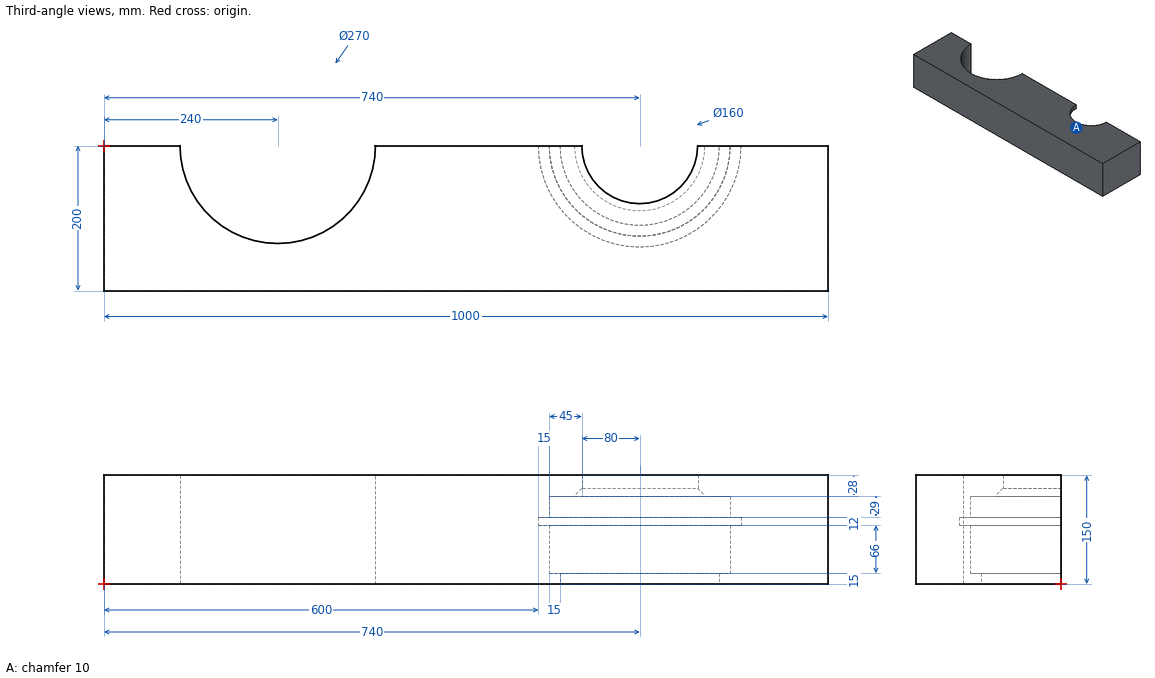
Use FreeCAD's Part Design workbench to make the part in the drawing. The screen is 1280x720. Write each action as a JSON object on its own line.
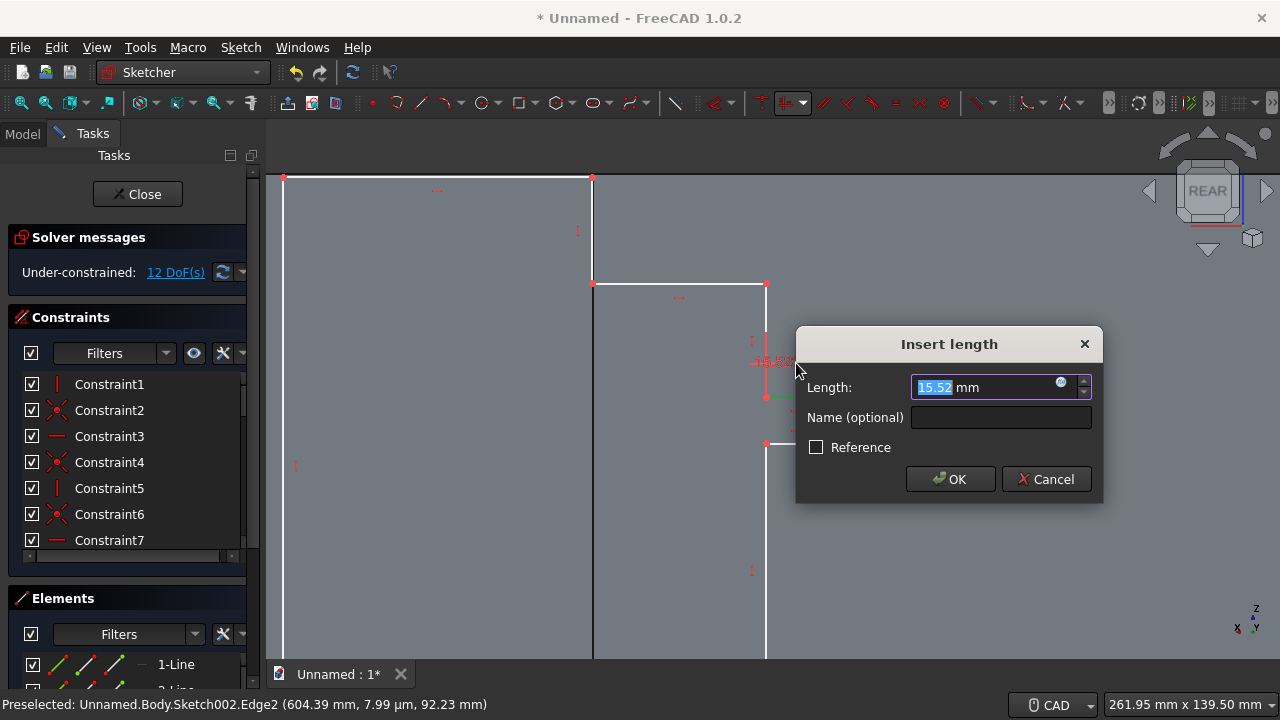
{"action": "type", "text": "15"}
{"action": "key", "text": "Return"}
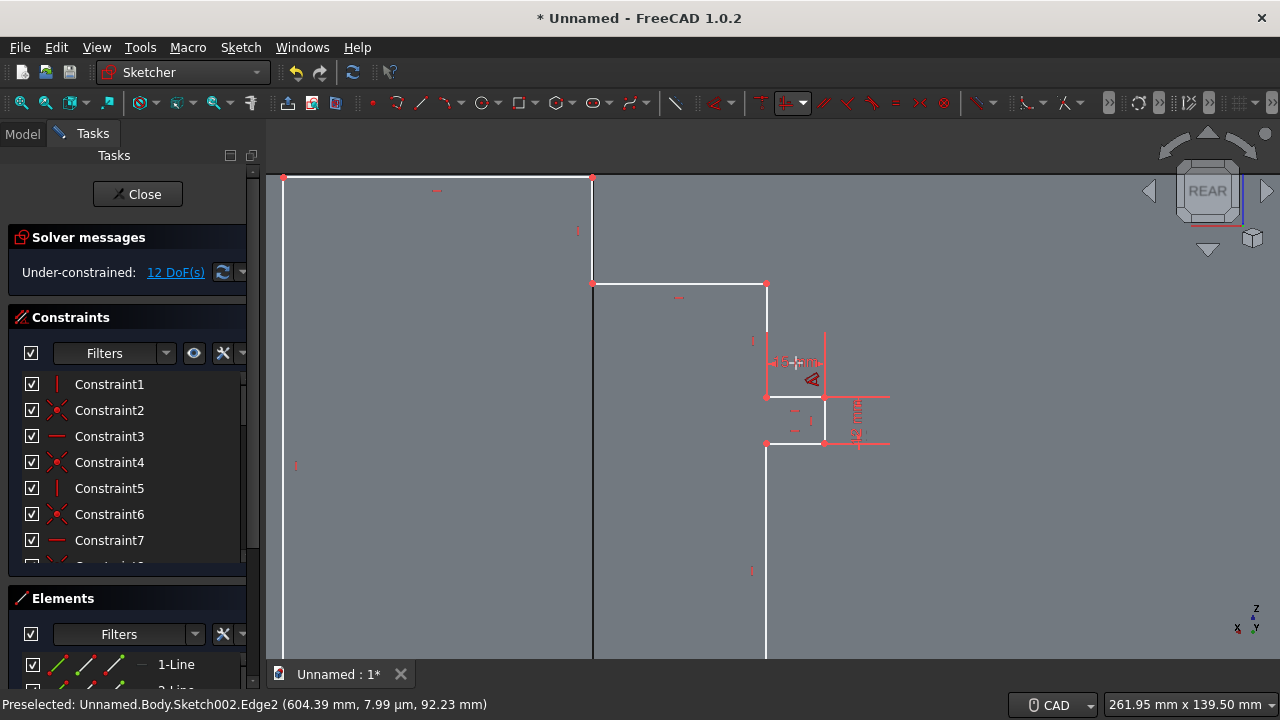
{"action": "left_click", "coordinate": [767, 363]}
{"action": "left_click", "coordinate": [801, 341]}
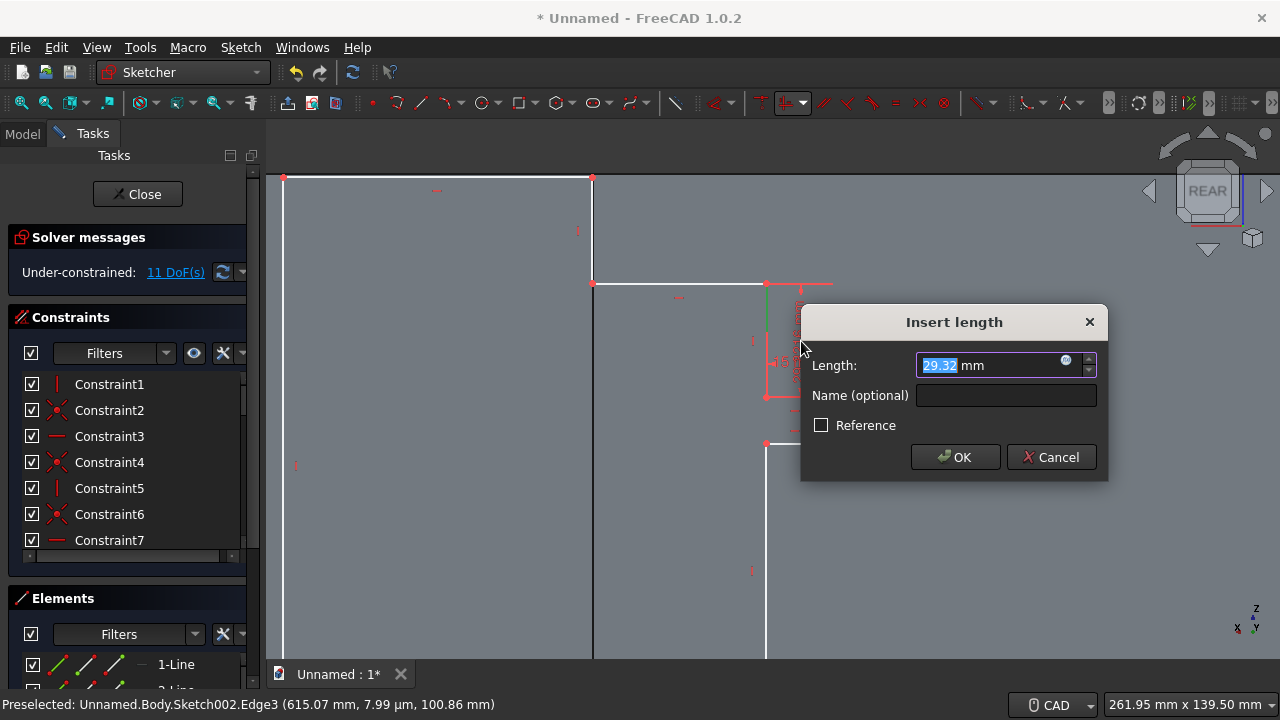
{"action": "type", "text": "29"}
{"action": "key", "text": "Return"}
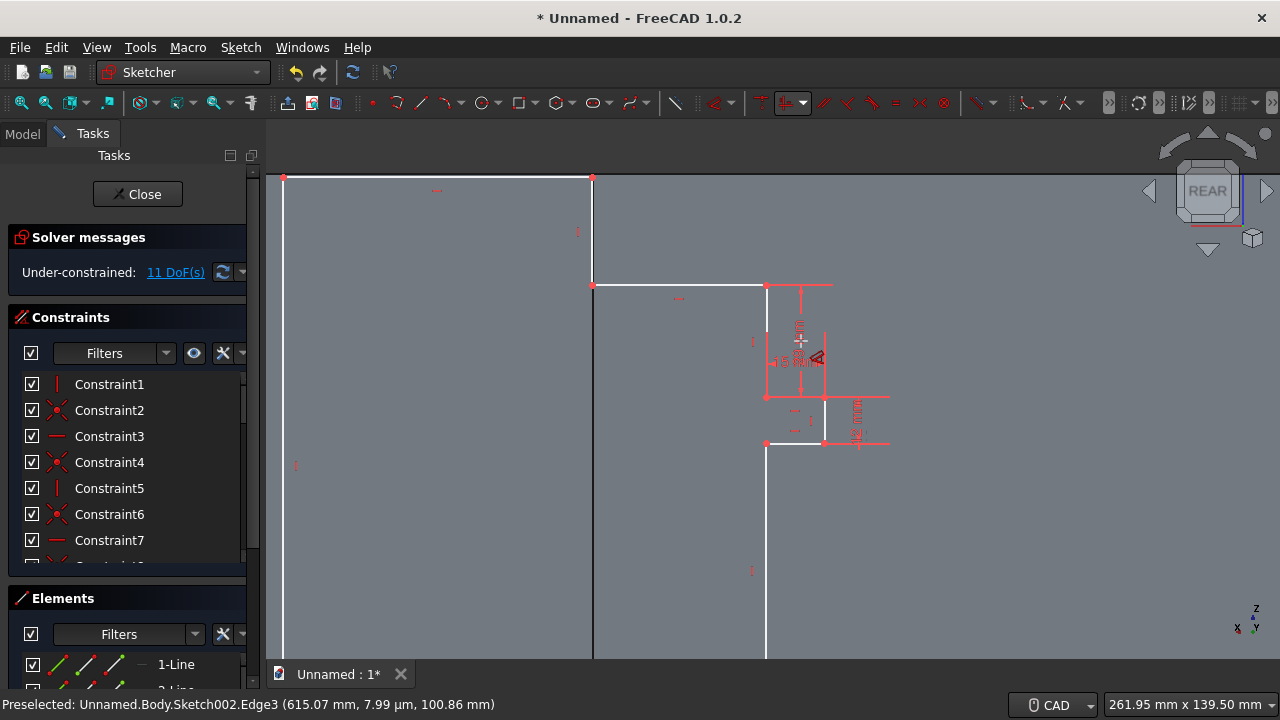
{"action": "left_click", "coordinate": [714, 285]}
{"action": "left_click", "coordinate": [680, 251]}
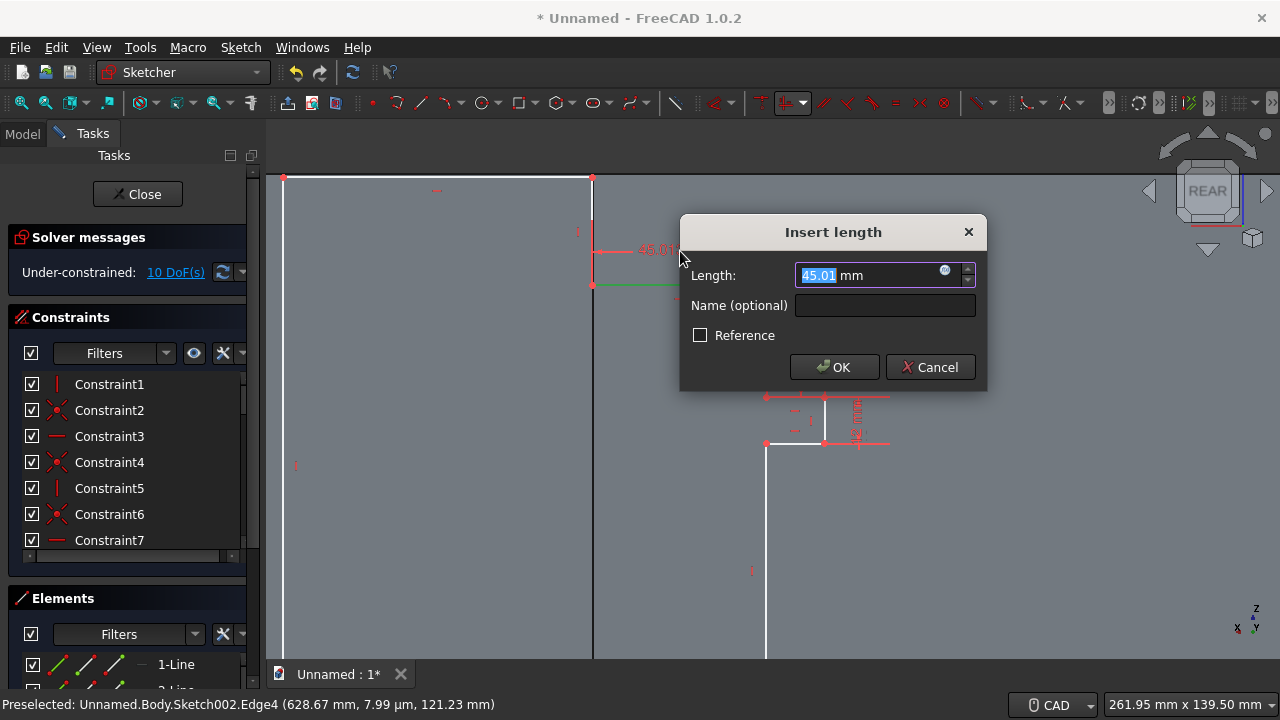
{"action": "type", "text": "45"}
{"action": "key", "text": "Return"}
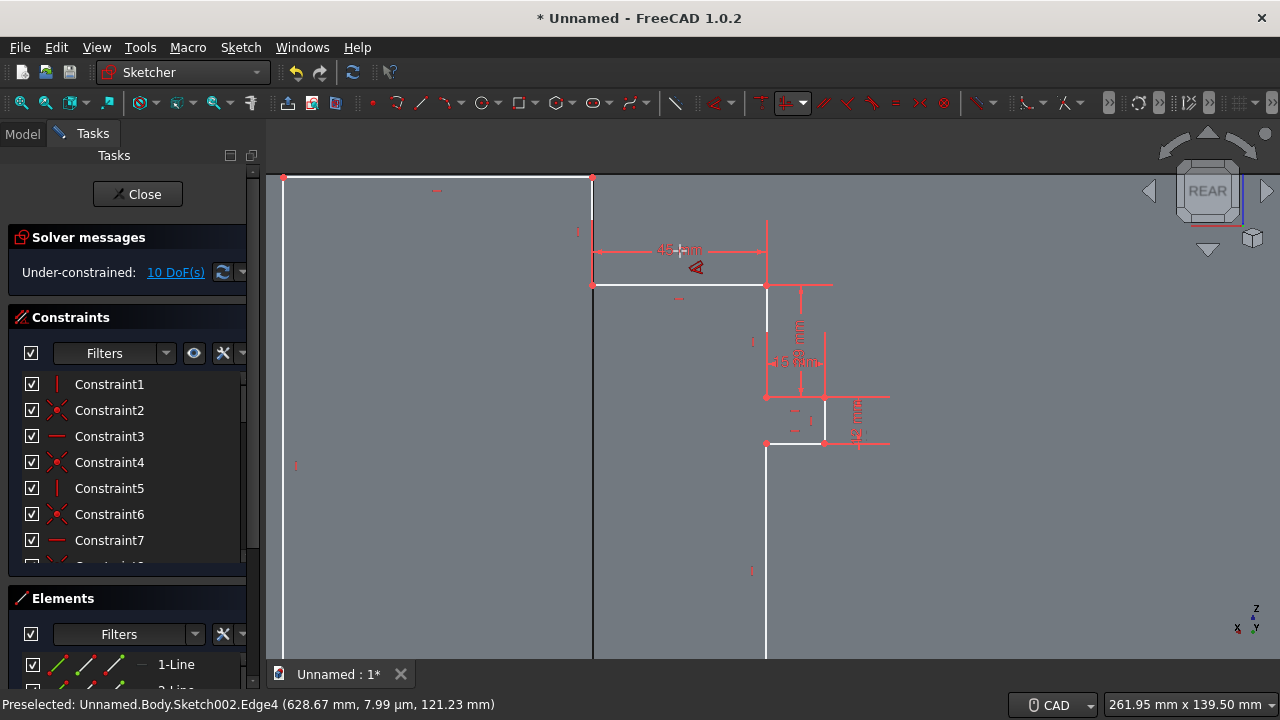
{"action": "left_click", "coordinate": [592, 253]}
{"action": "left_click", "coordinate": [626, 231]}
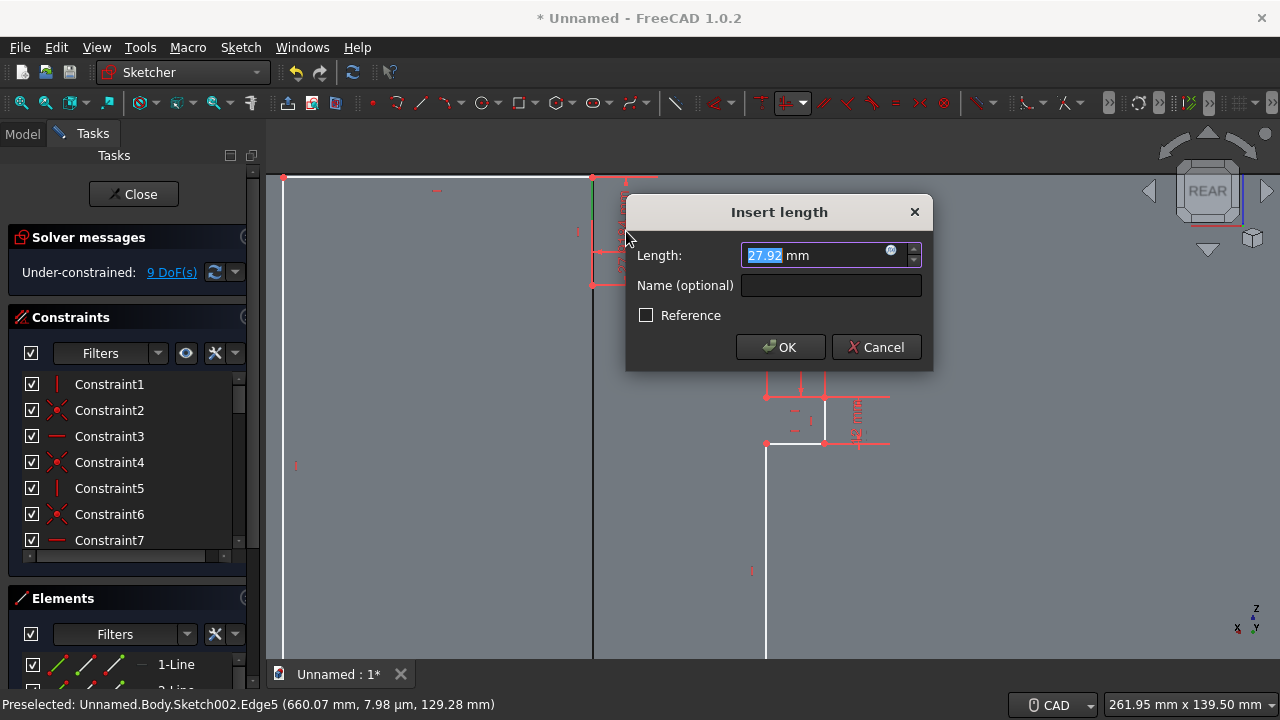
{"action": "type", "text": "28"}
{"action": "key", "text": "Return"}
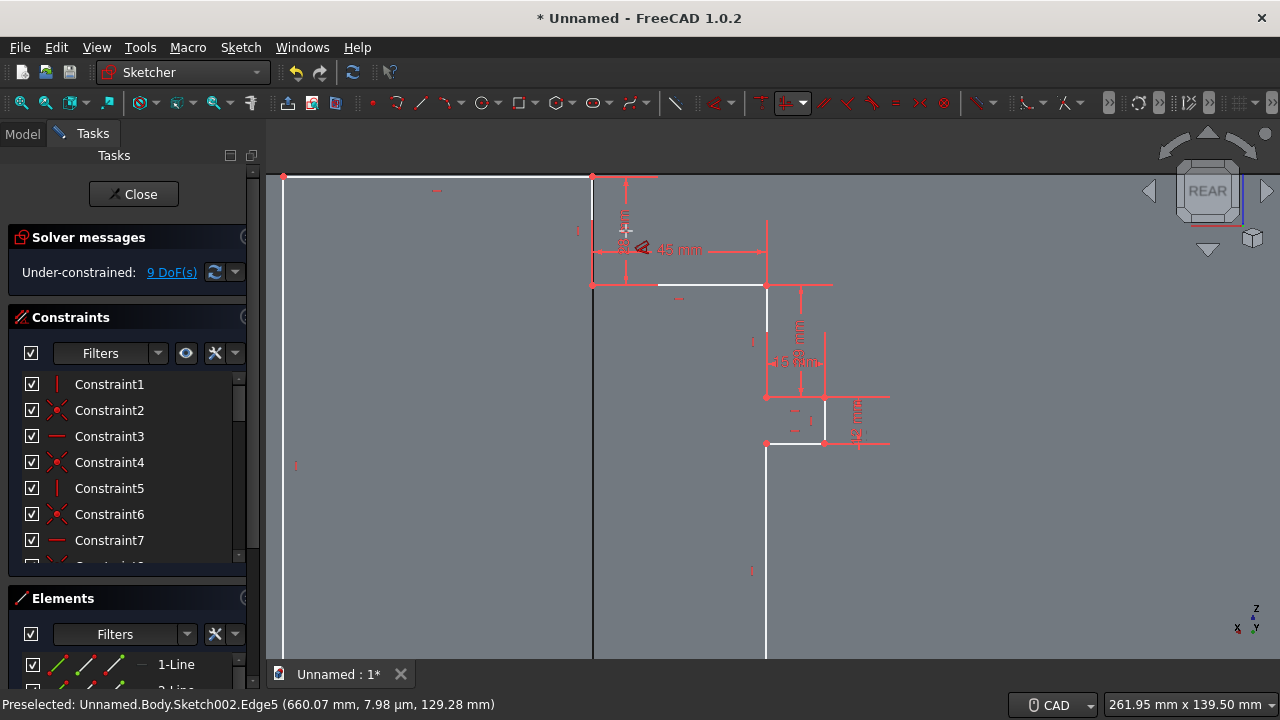
{"action": "left_click", "coordinate": [500, 177]}
{"action": "left_click", "coordinate": [443, 211]}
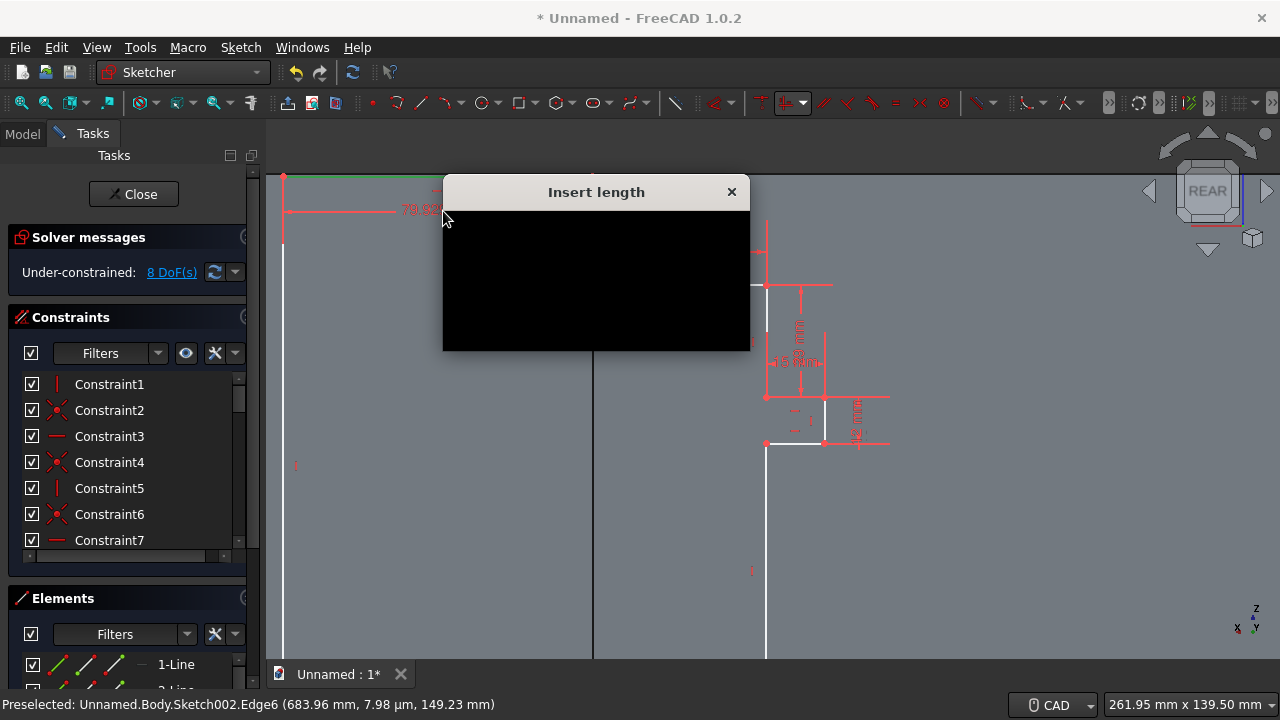
{"action": "type", "text": "80"}
{"action": "key", "text": "Return"}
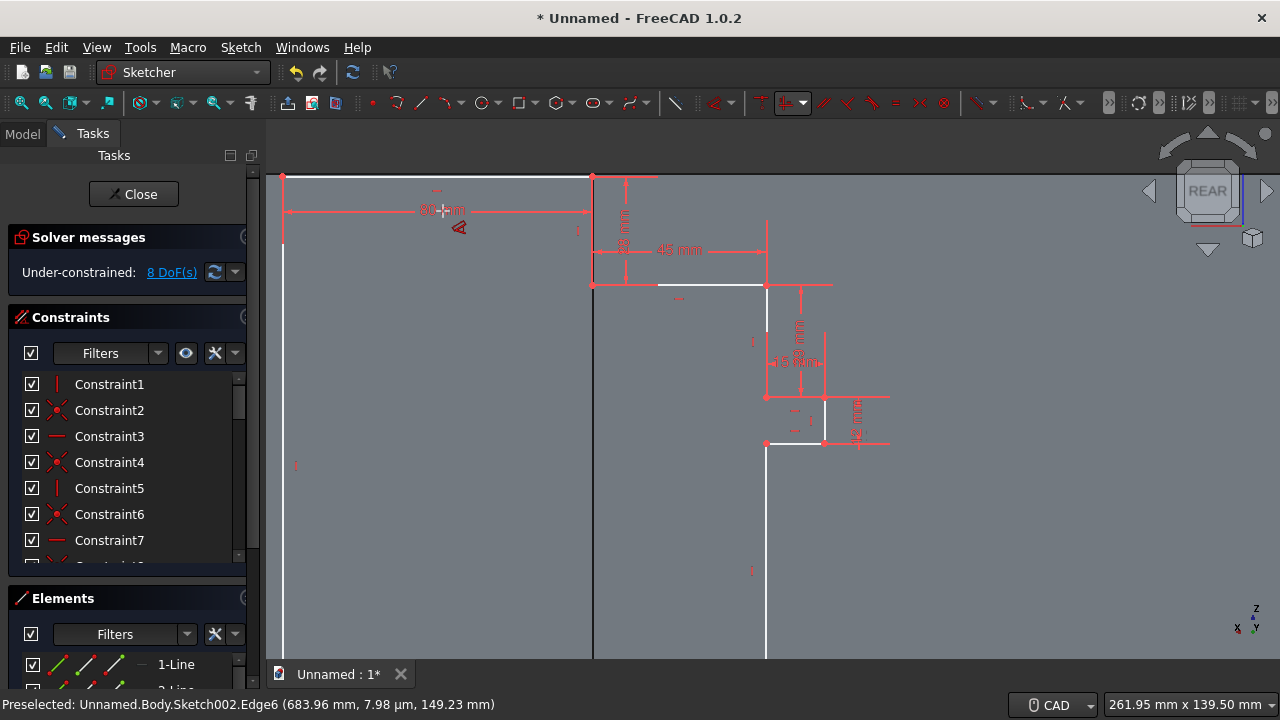
{"action": "scroll", "coordinate": [827, 422], "scroll_direction": "down", "scroll_amount": 4}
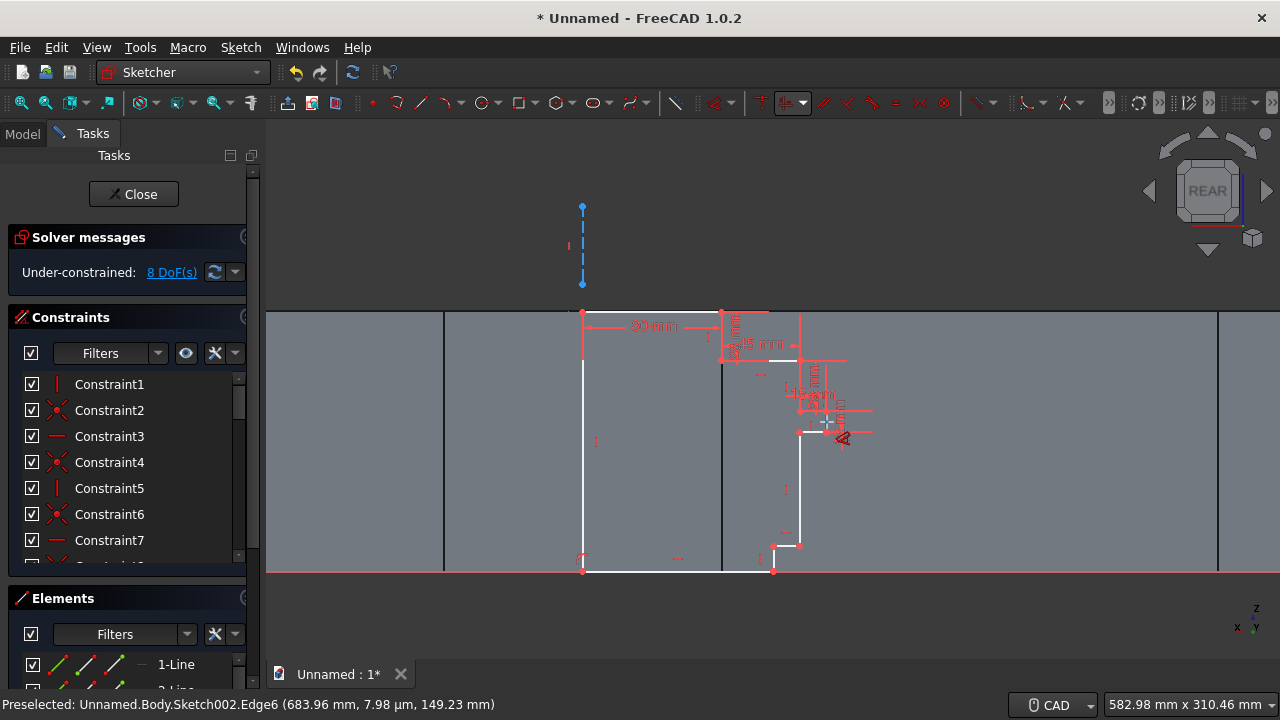
{"action": "scroll", "coordinate": [774, 564], "scroll_direction": "up", "scroll_amount": 3}